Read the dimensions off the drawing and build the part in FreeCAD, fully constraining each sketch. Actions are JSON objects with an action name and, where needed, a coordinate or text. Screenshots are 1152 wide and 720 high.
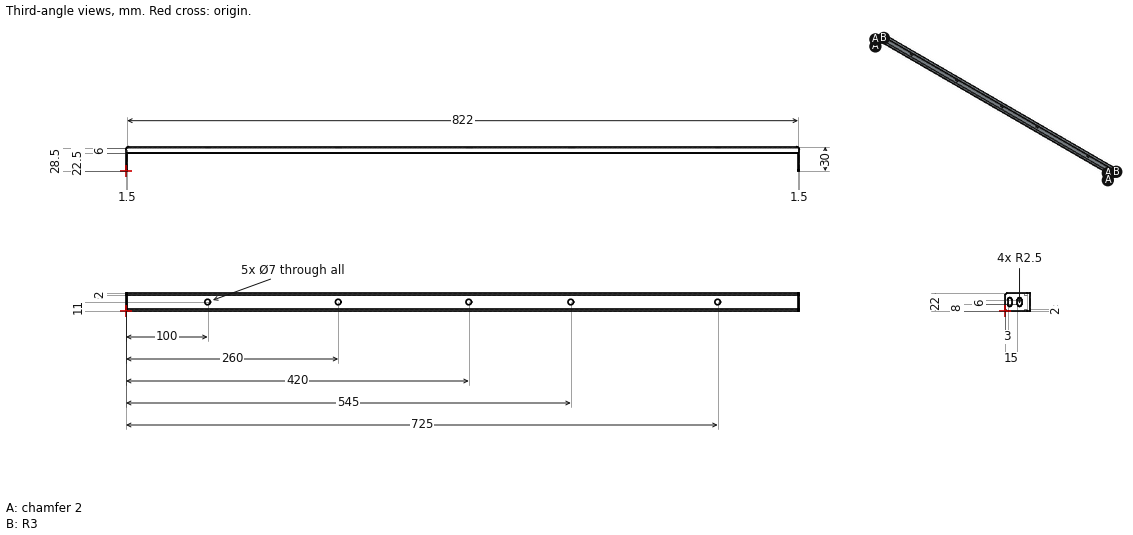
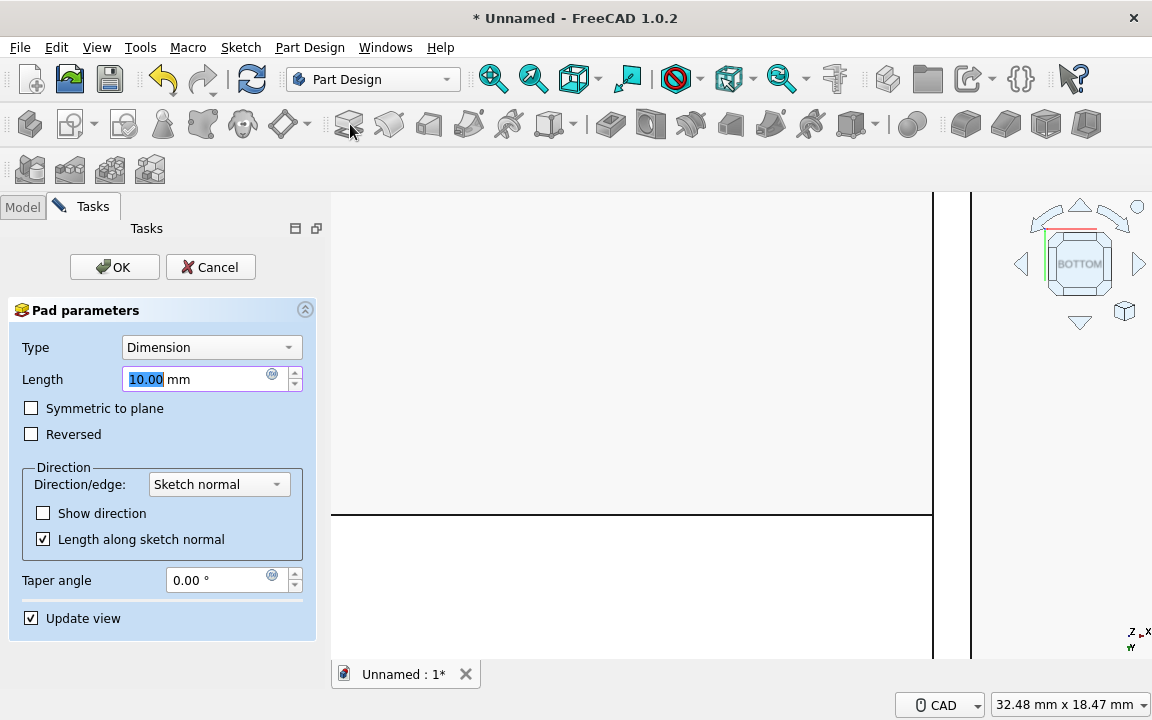
{"action": "type", "text": "2"}
{"action": "key", "text": "Tab"}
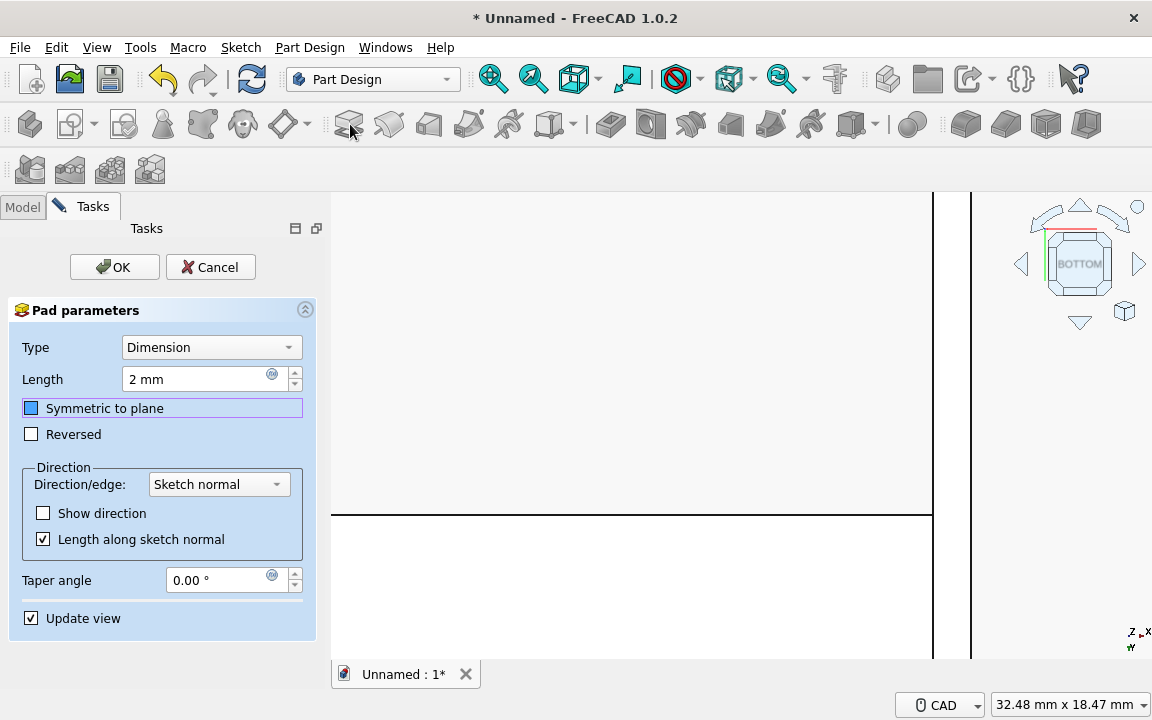
{"action": "left_click", "coordinate": [30, 434]}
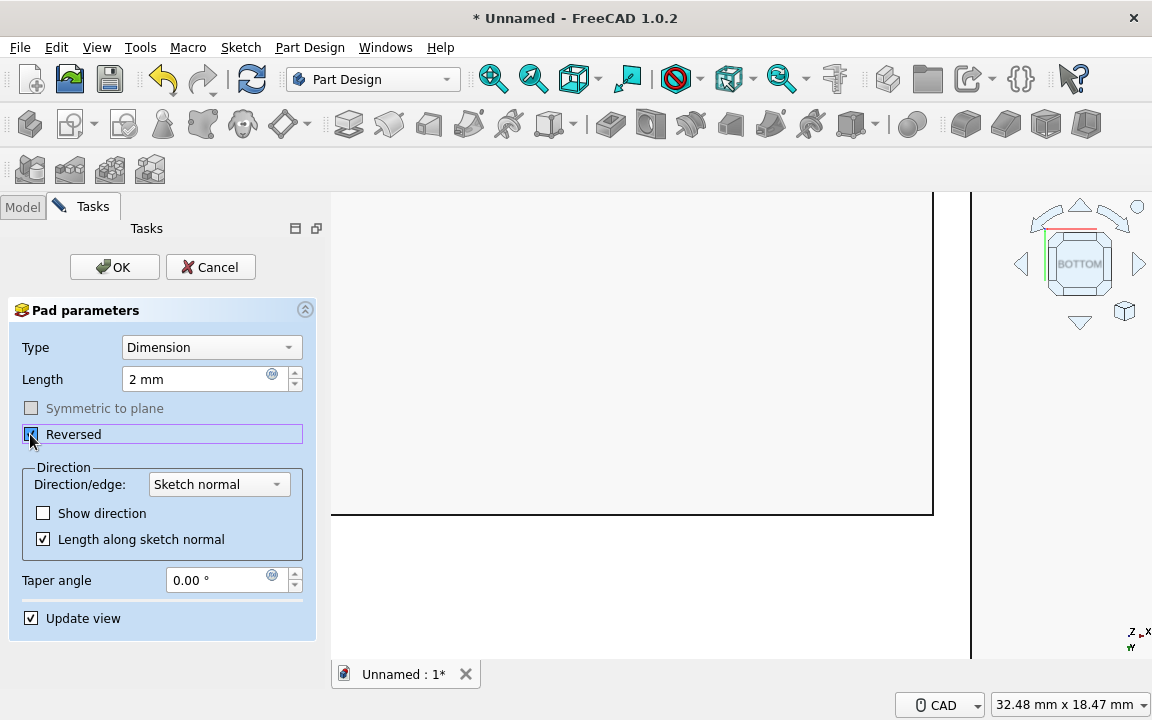
{"action": "left_click", "coordinate": [115, 267]}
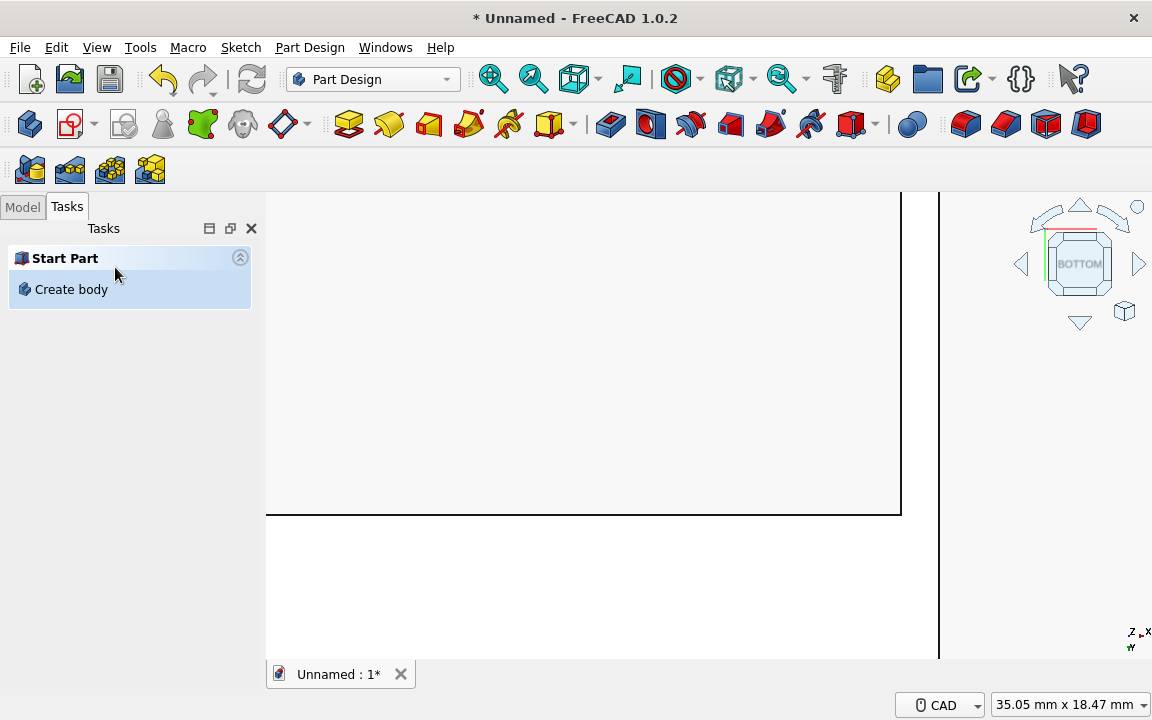
{"action": "left_click", "coordinate": [494, 80]}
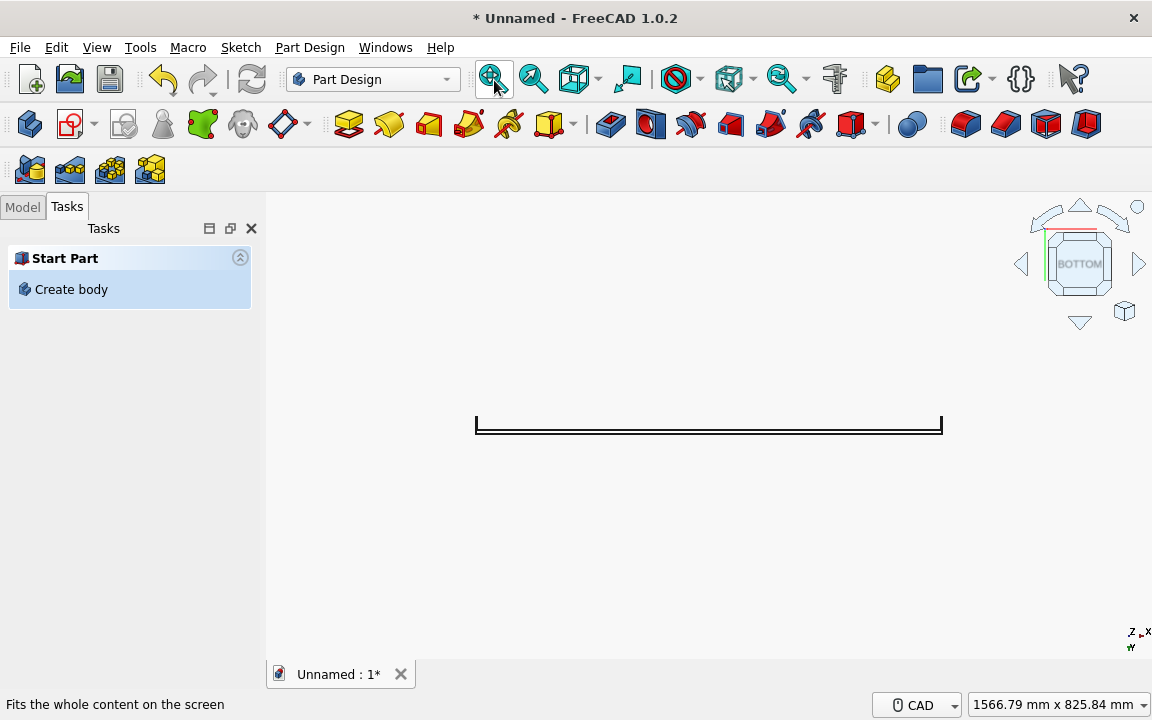
{"action": "left_click", "coordinate": [70, 124]}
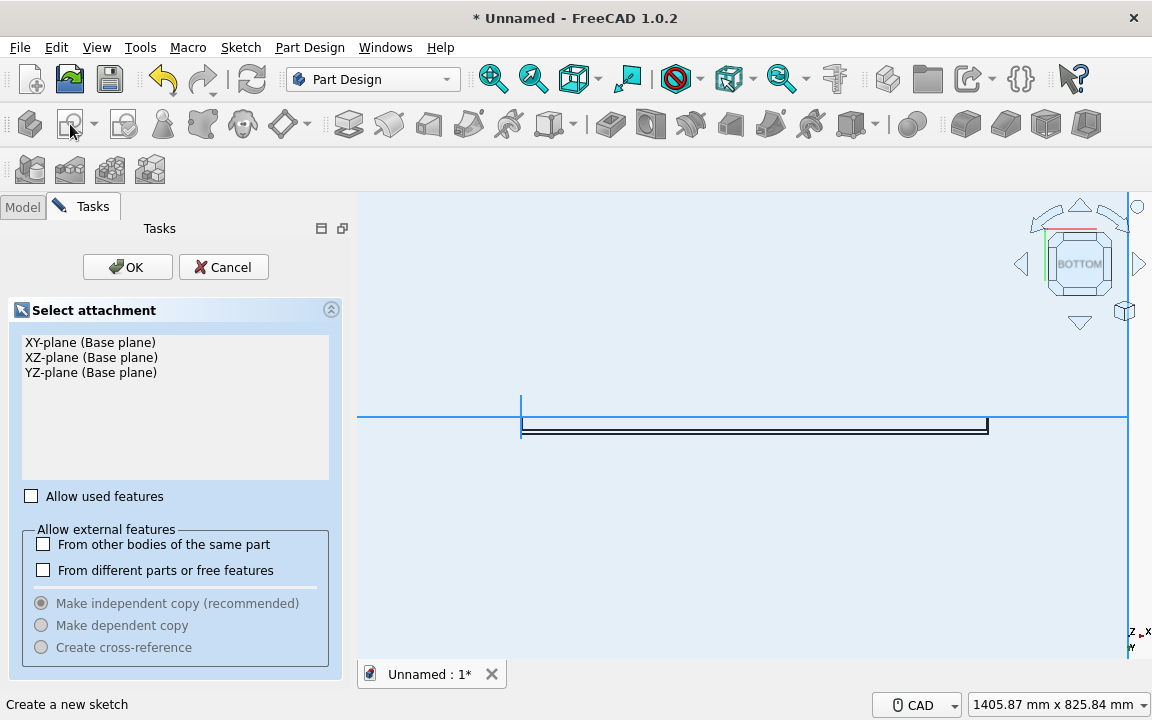
{"action": "left_click", "coordinate": [82, 372]}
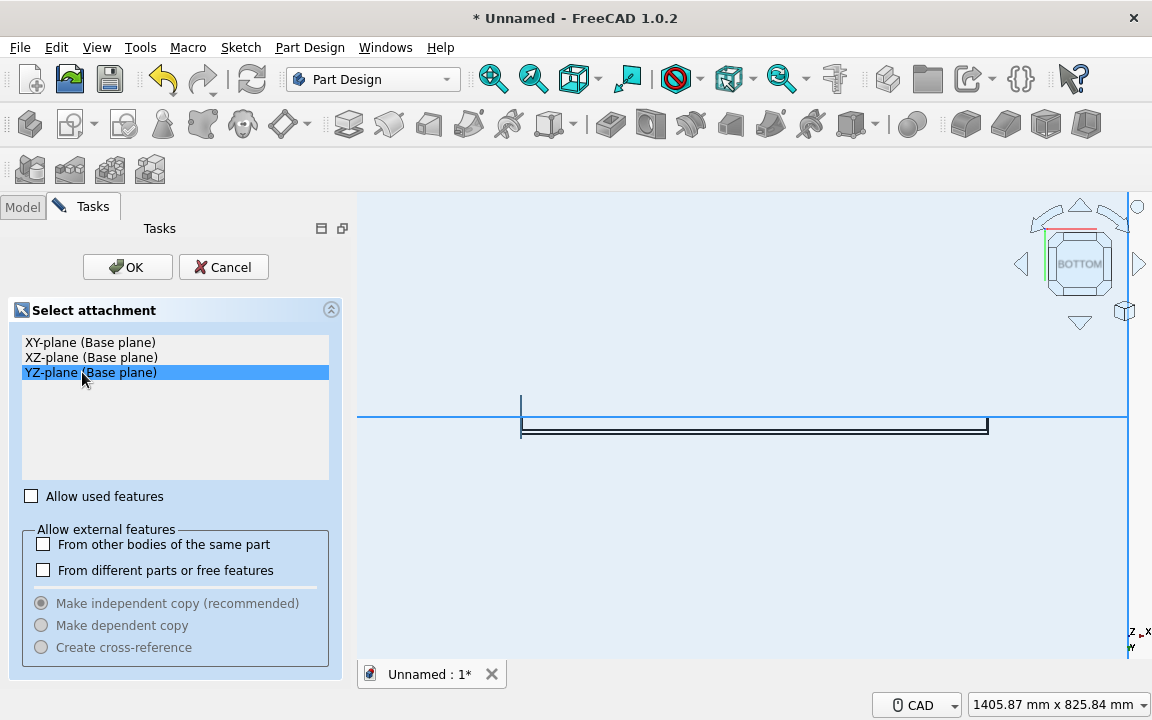
{"action": "left_click", "coordinate": [128, 267]}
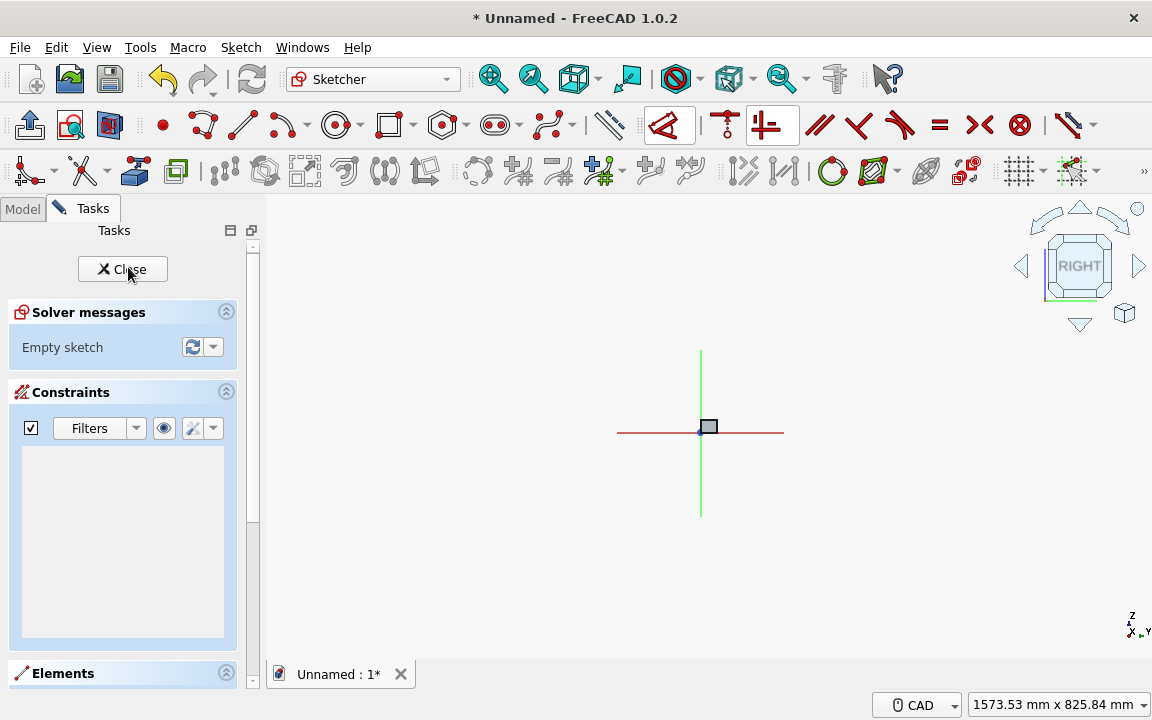
{"action": "left_click", "coordinate": [110, 126]}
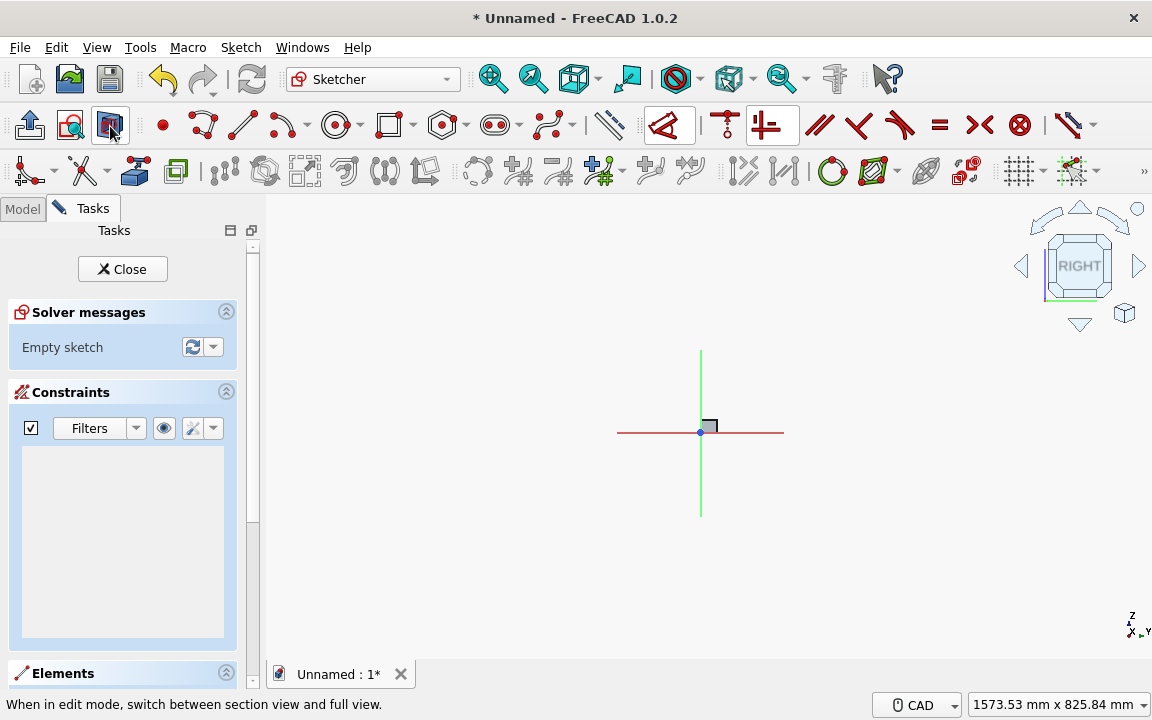
{"action": "scroll", "coordinate": [710, 428], "scroll_direction": "up", "scroll_amount": 15}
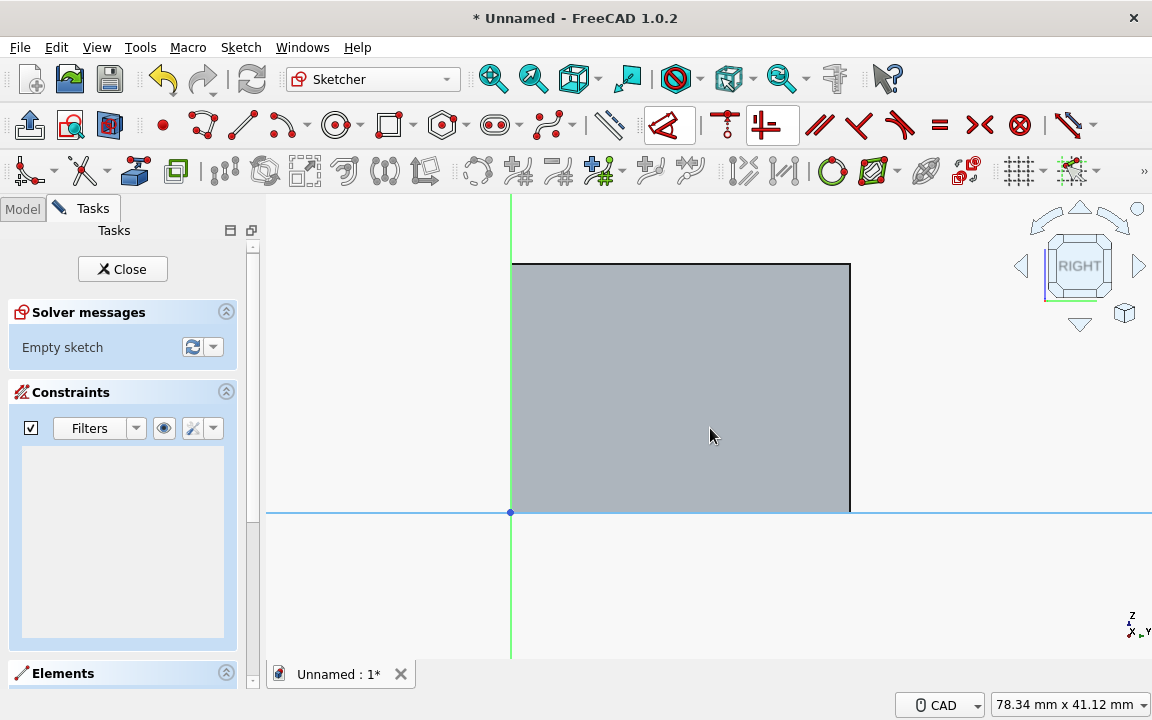
{"action": "scroll", "coordinate": [590, 405], "scroll_direction": "up", "scroll_amount": 2}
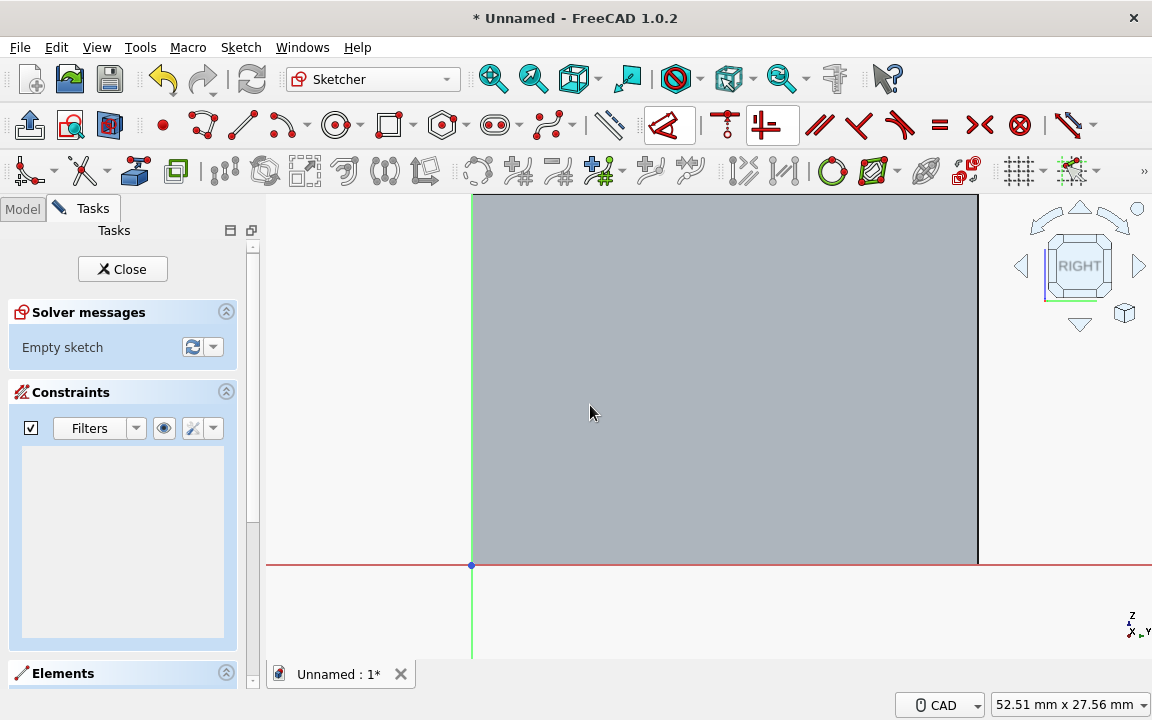
{"action": "left_click", "coordinate": [496, 126]}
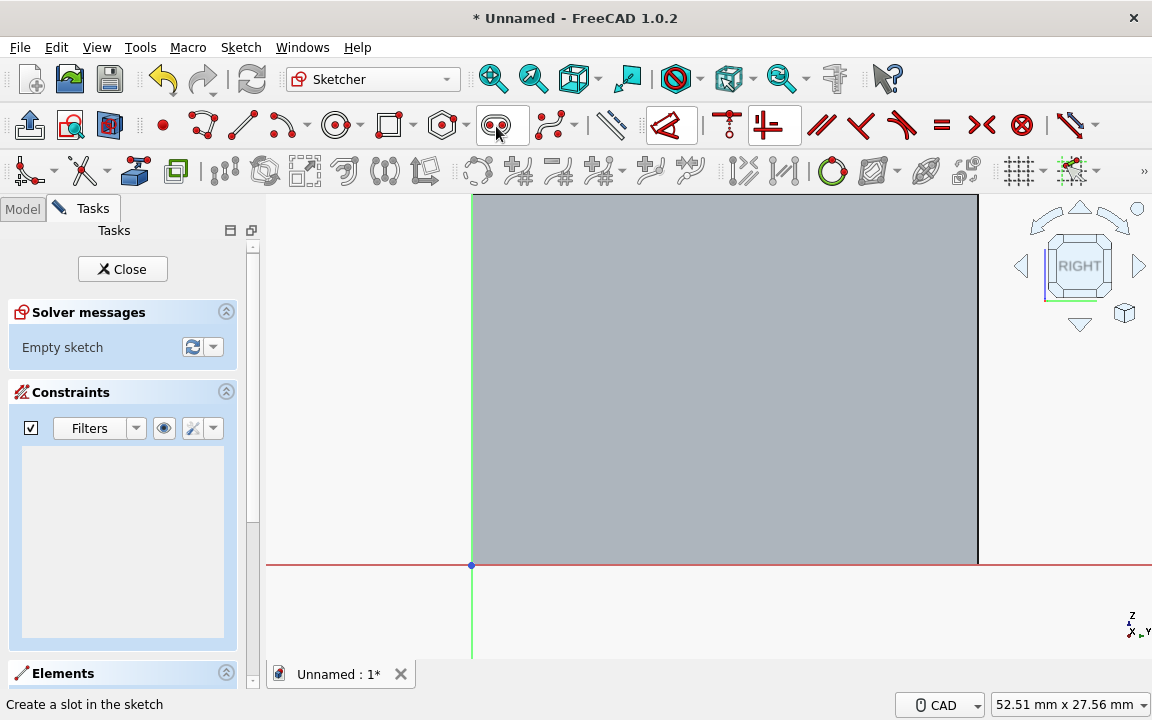
{"action": "left_click", "coordinate": [767, 430]}